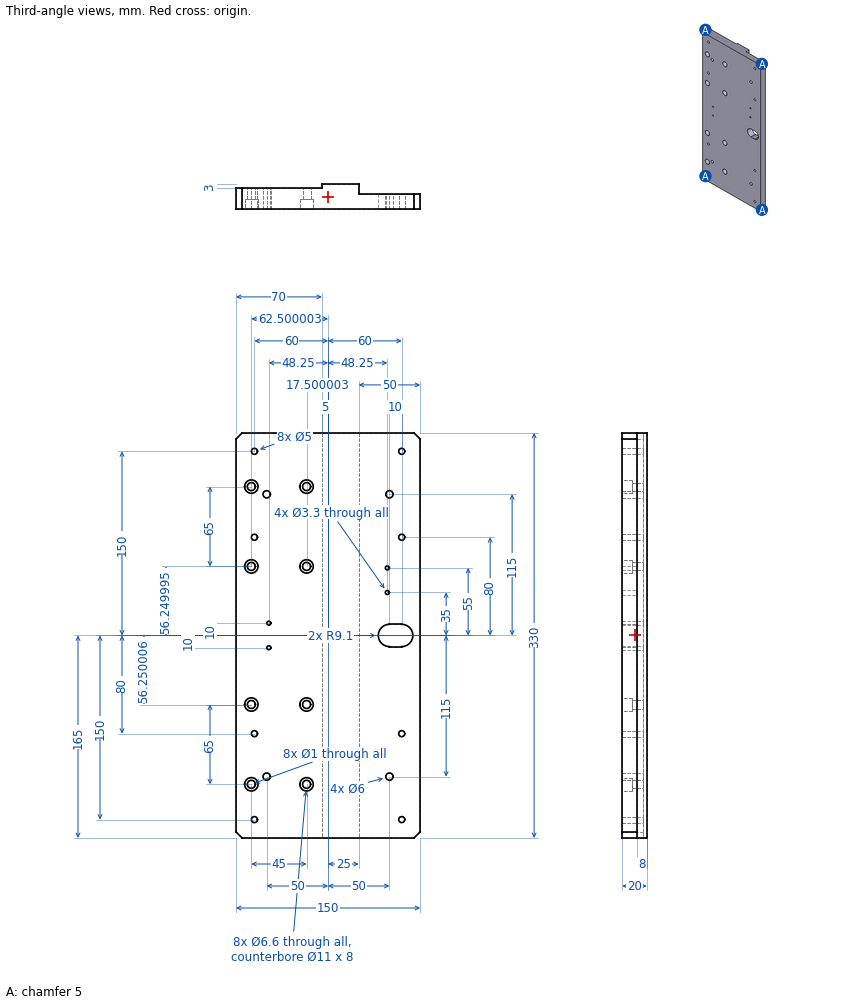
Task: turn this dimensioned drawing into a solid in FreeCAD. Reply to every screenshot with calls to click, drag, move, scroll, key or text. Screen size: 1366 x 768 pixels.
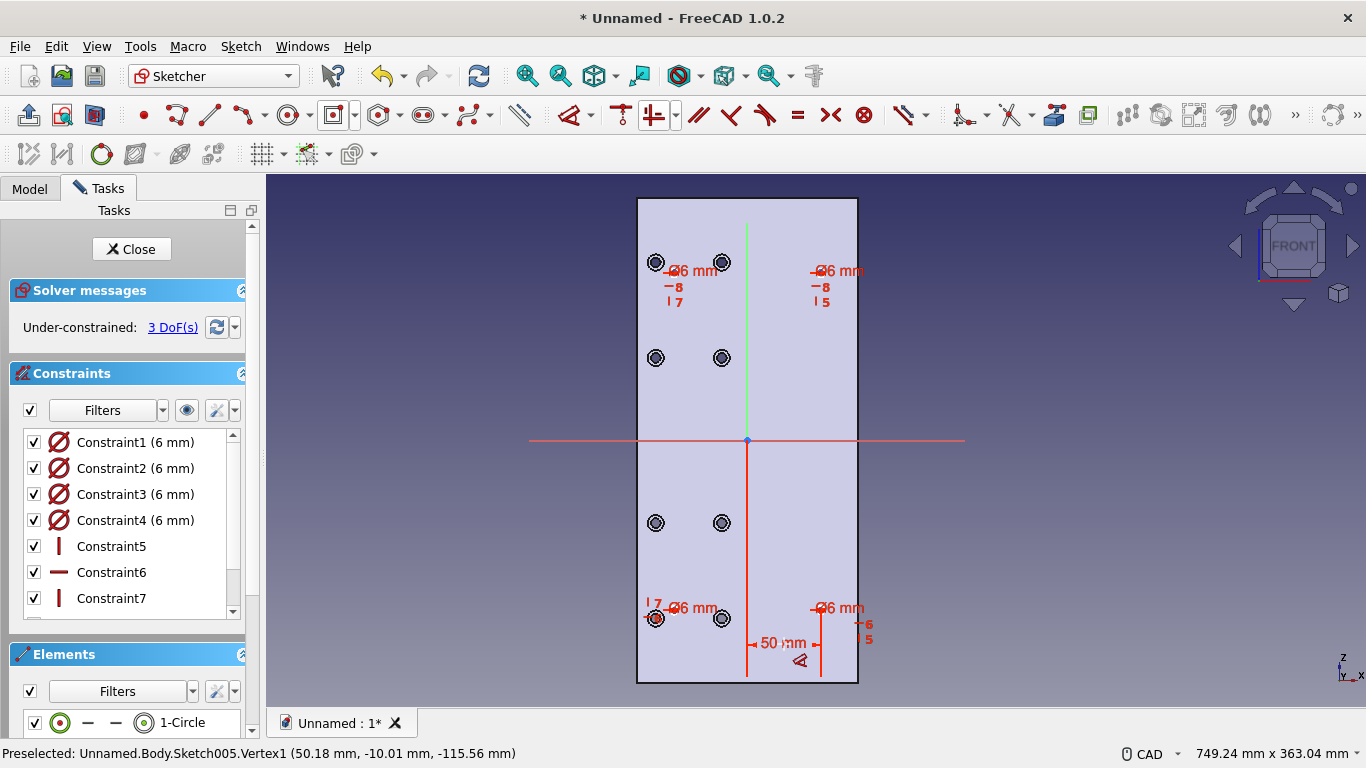
click(674, 610)
click(711, 644)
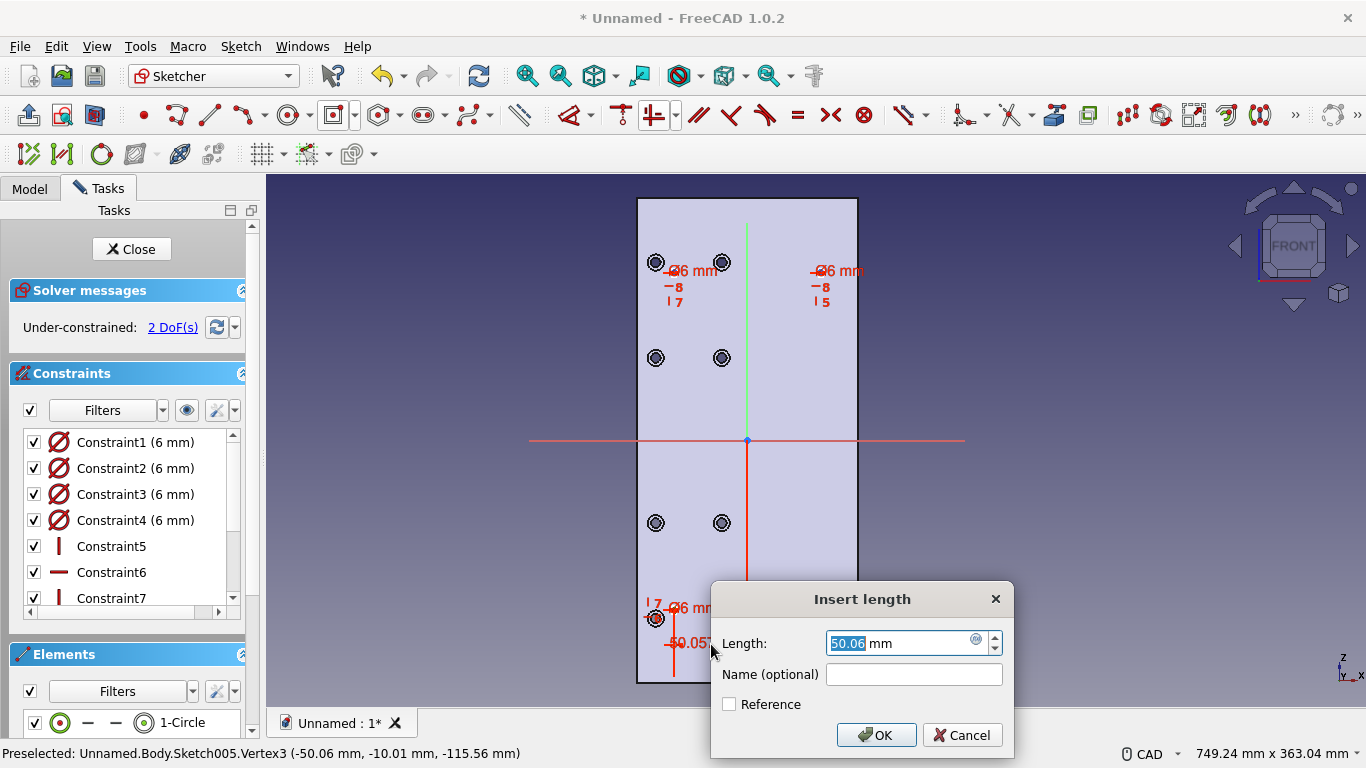
text(50)
key(Return)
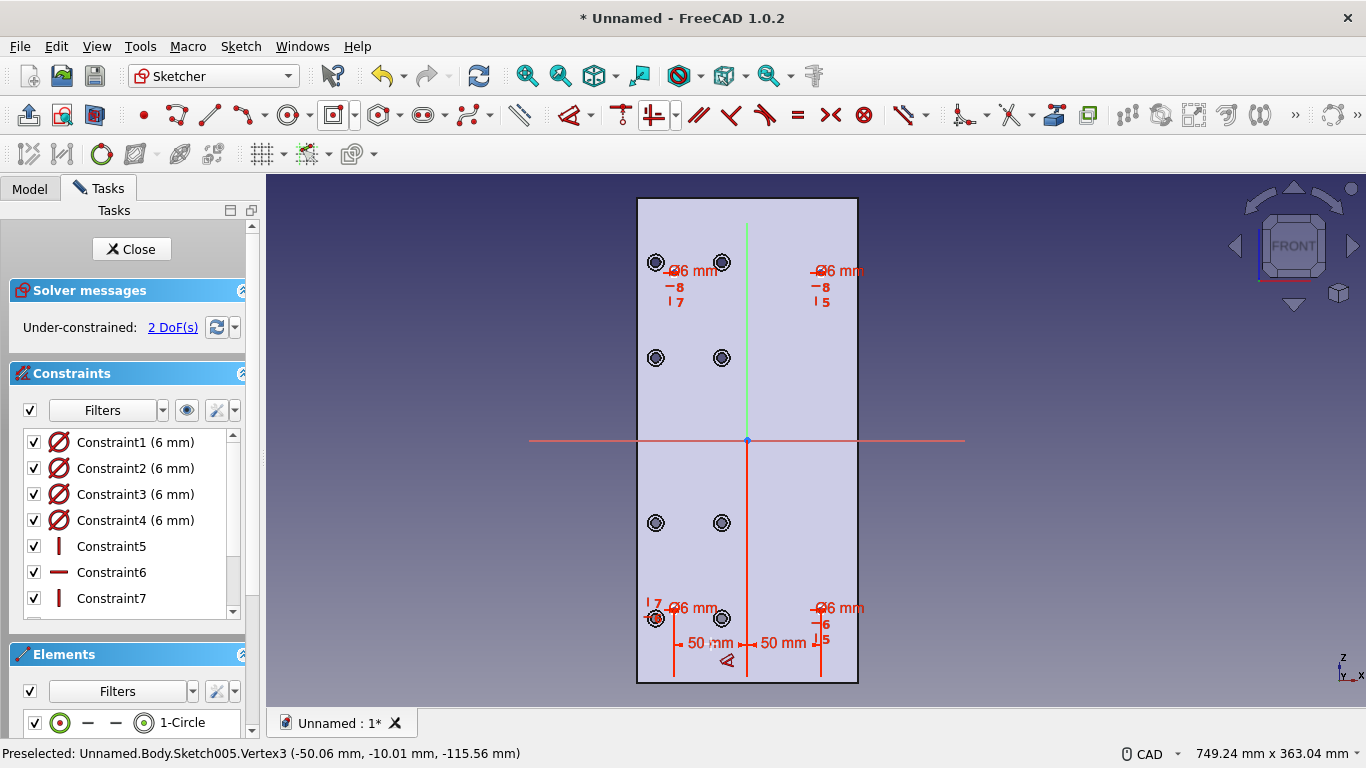
click(821, 610)
click(855, 525)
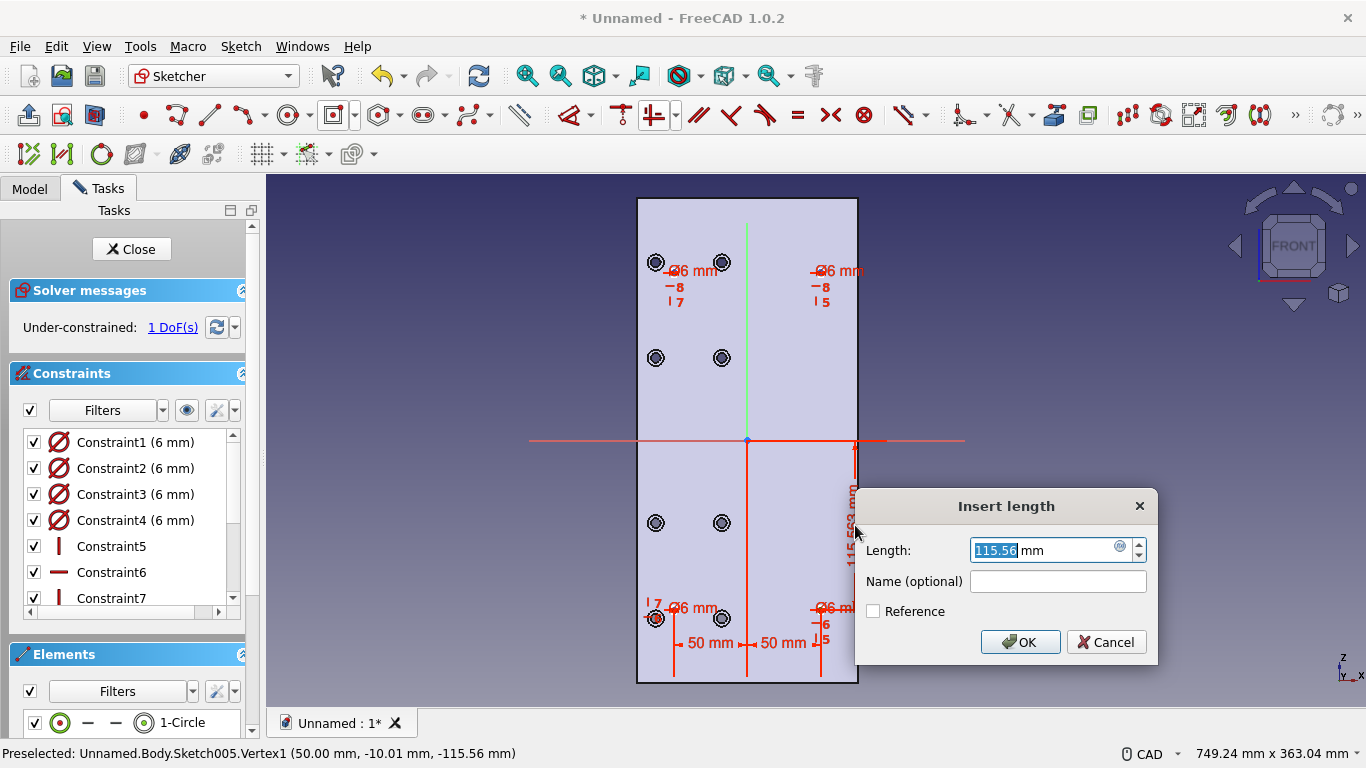
text(115)
key(Return)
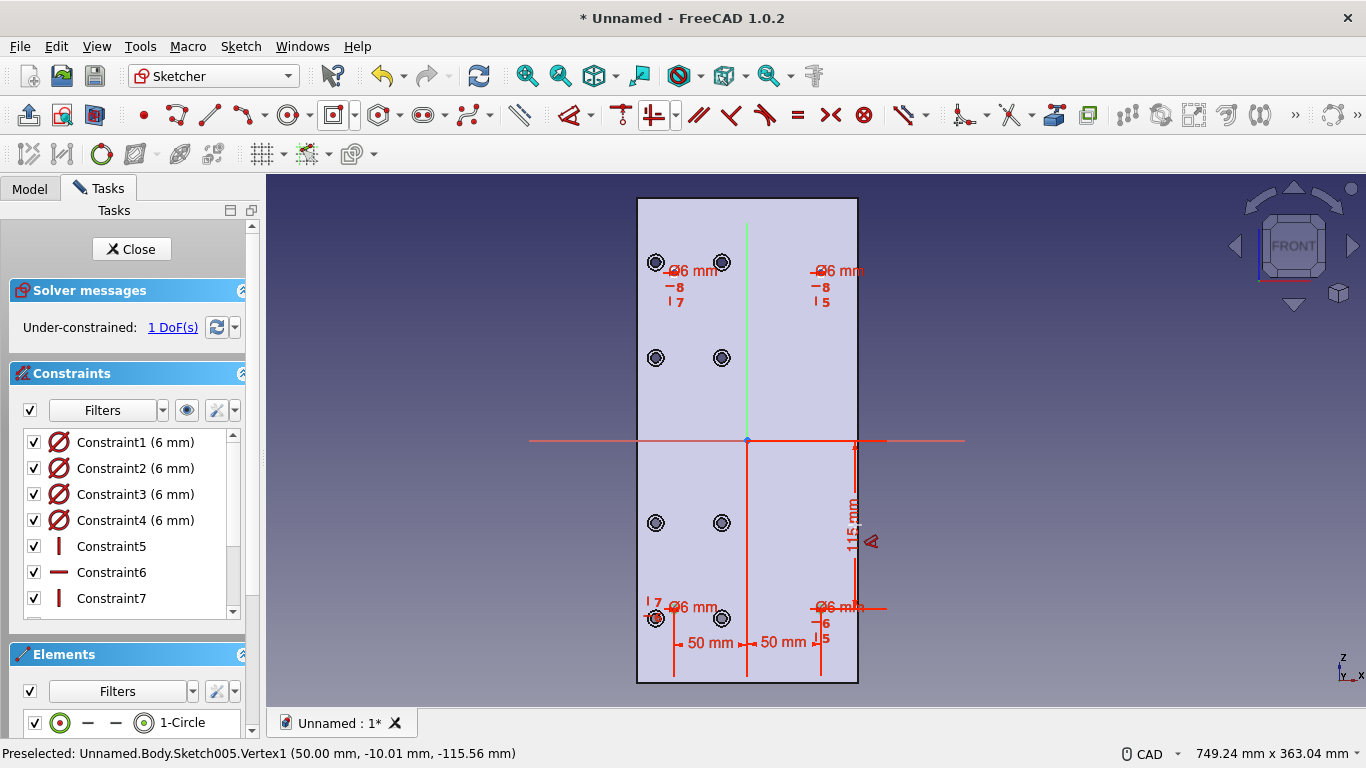
click(821, 273)
click(855, 357)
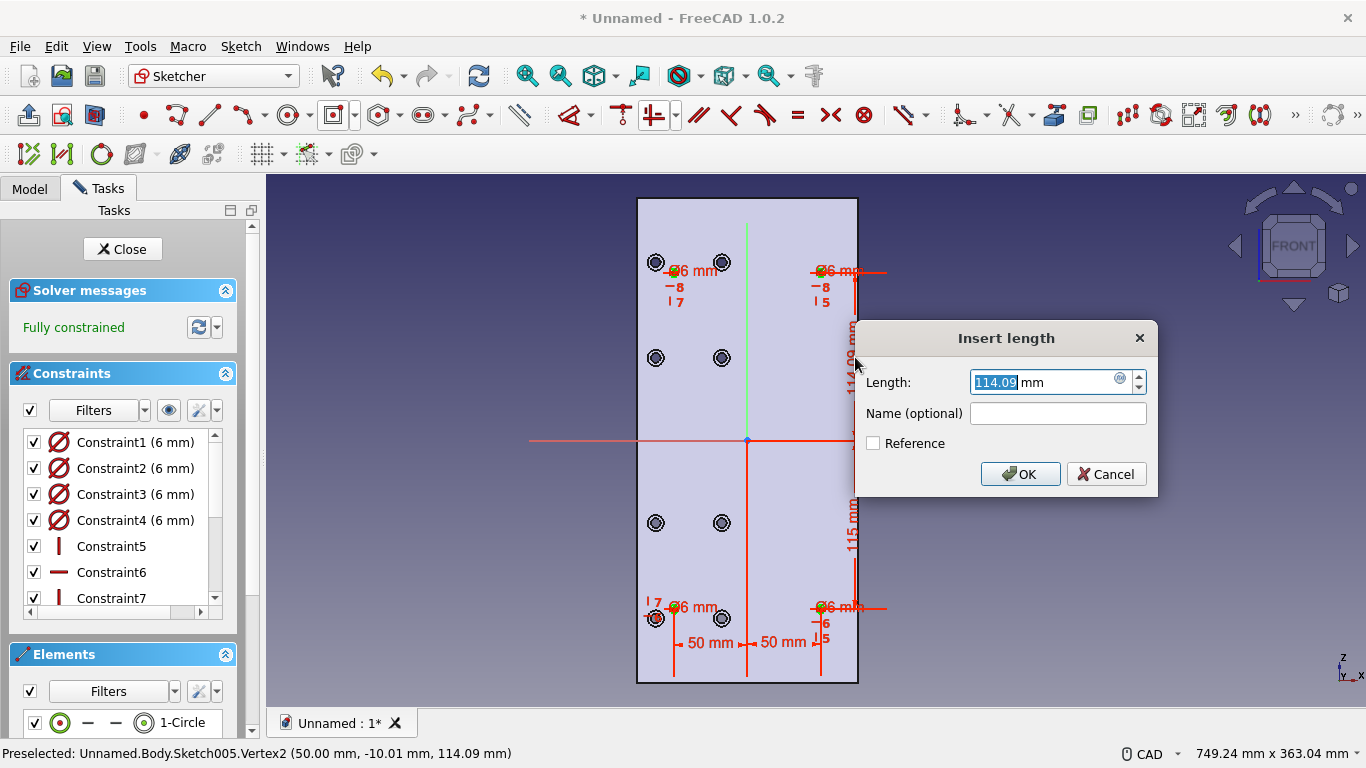
text(115)
key(Return)
key(Escape)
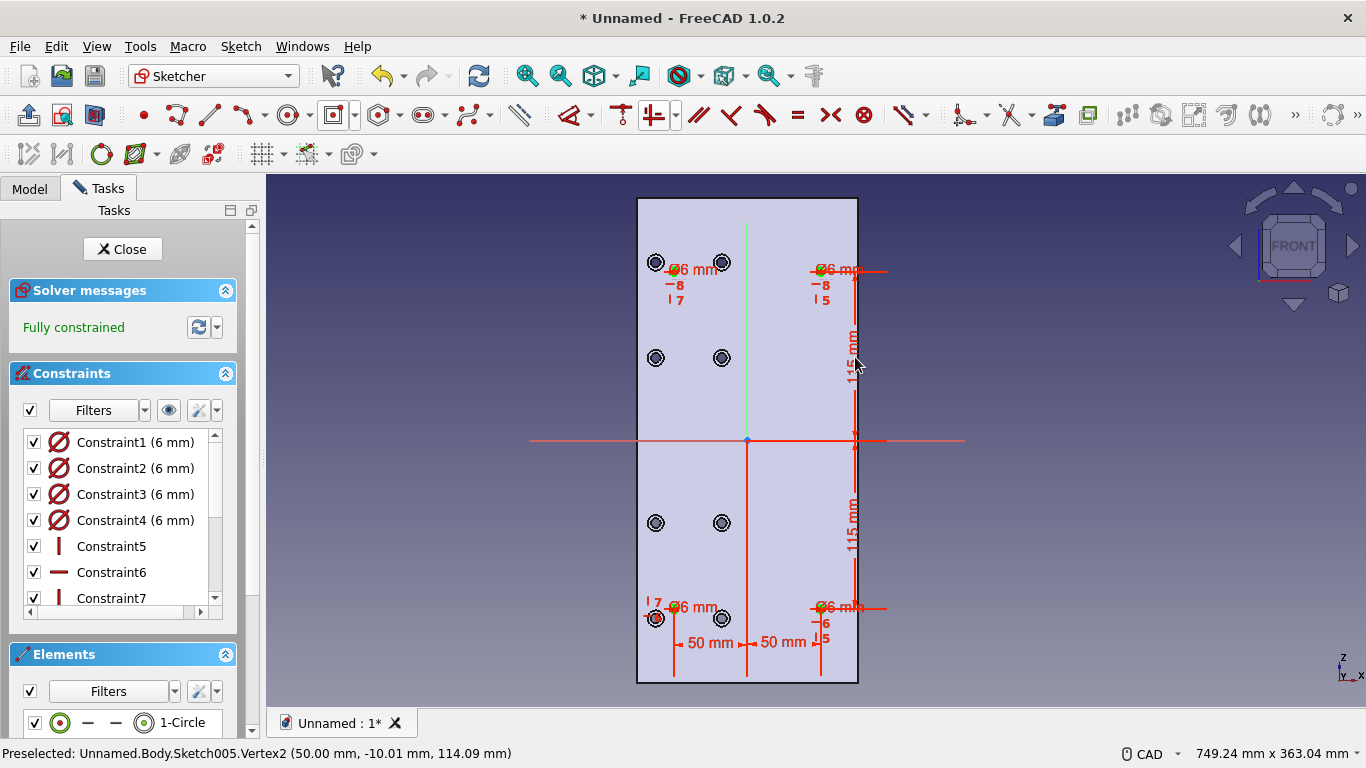
click(123, 249)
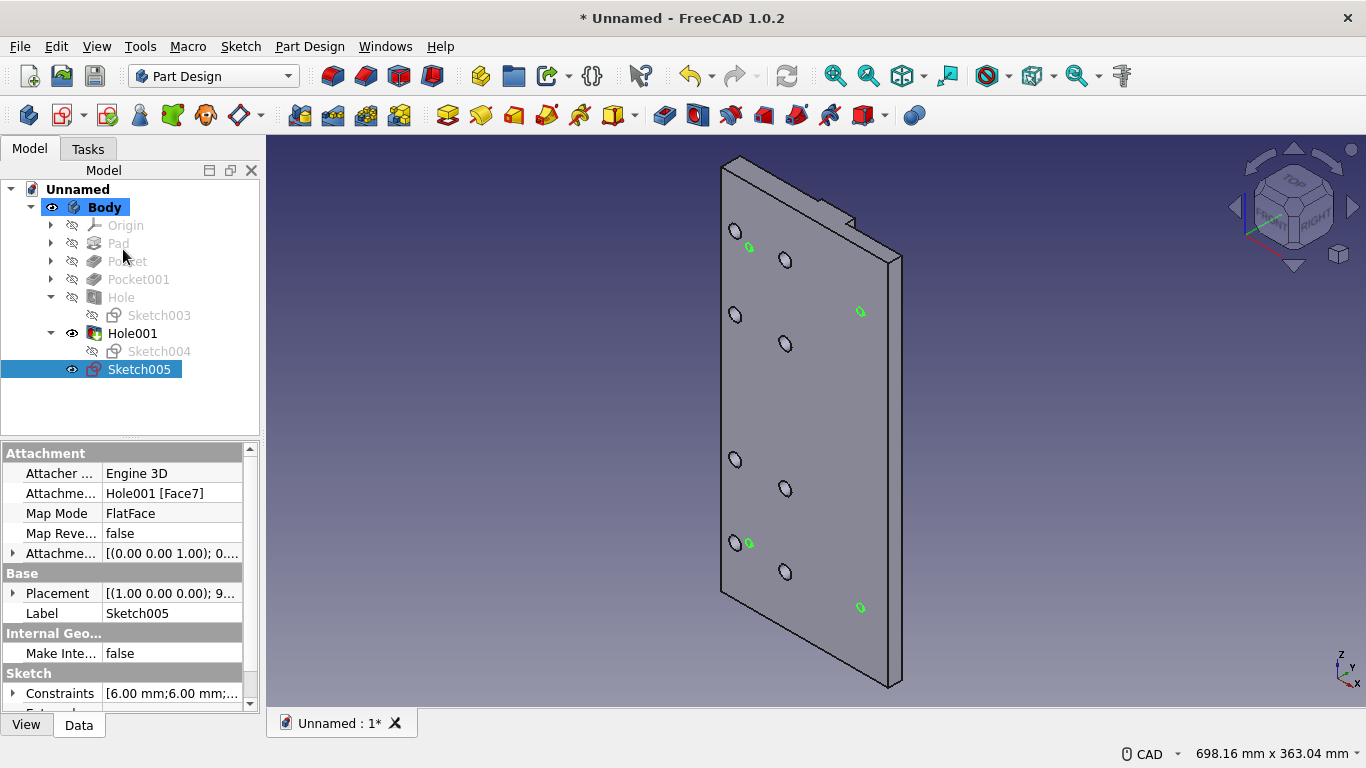
click(665, 116)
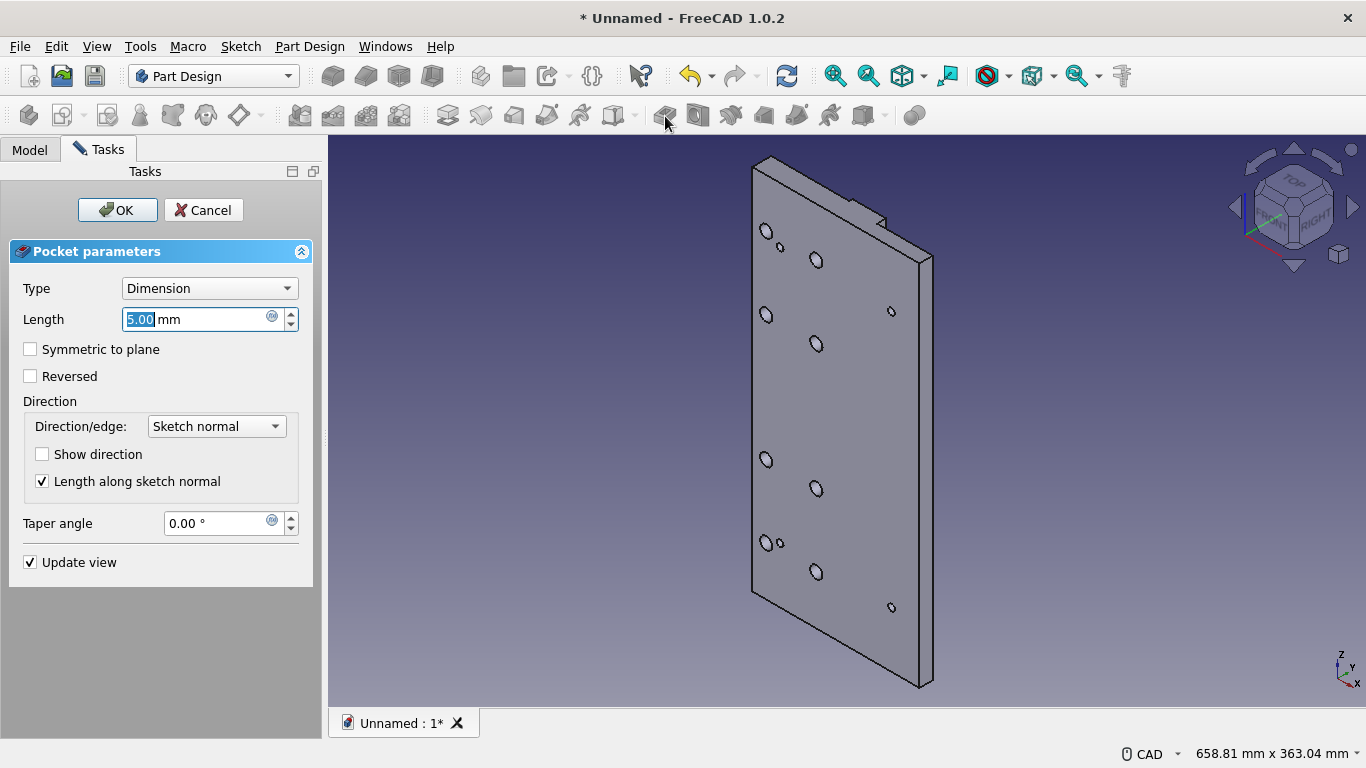
click(210, 288)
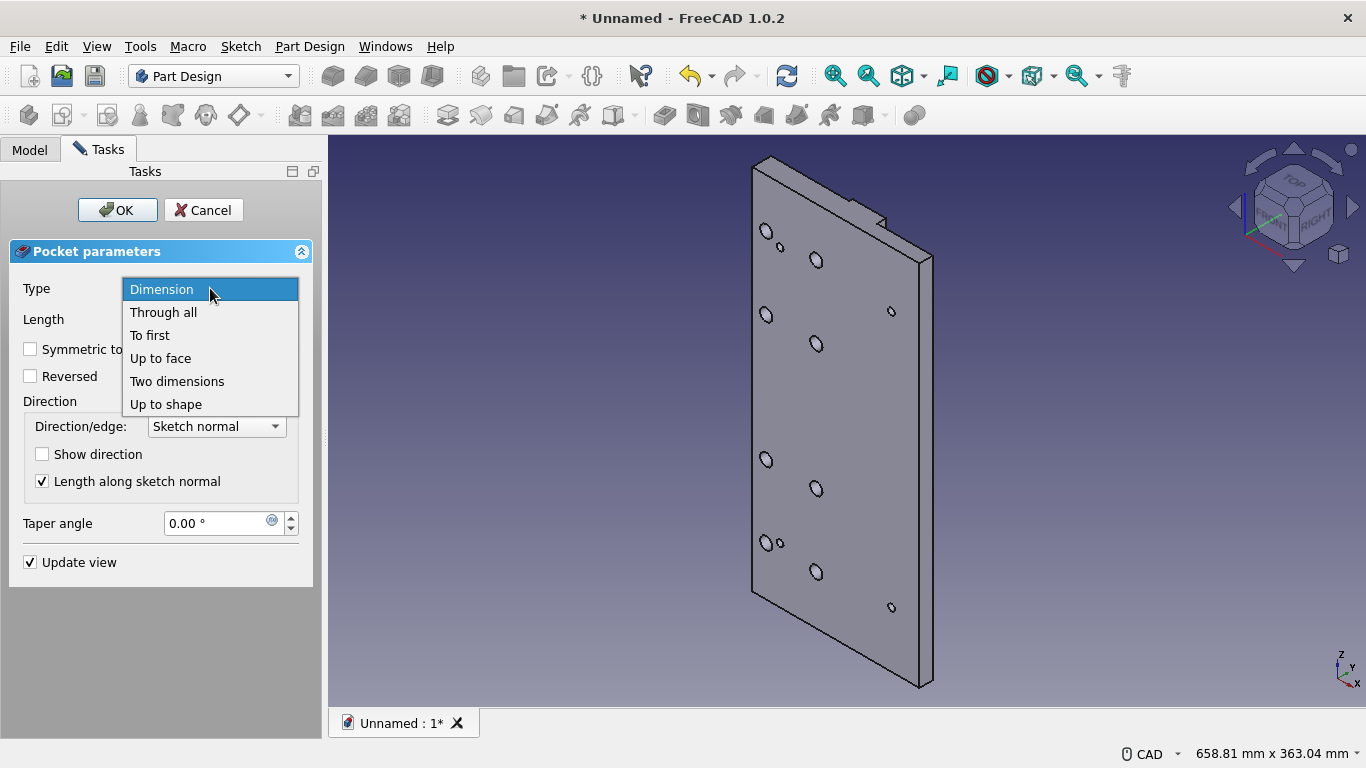
click(208, 312)